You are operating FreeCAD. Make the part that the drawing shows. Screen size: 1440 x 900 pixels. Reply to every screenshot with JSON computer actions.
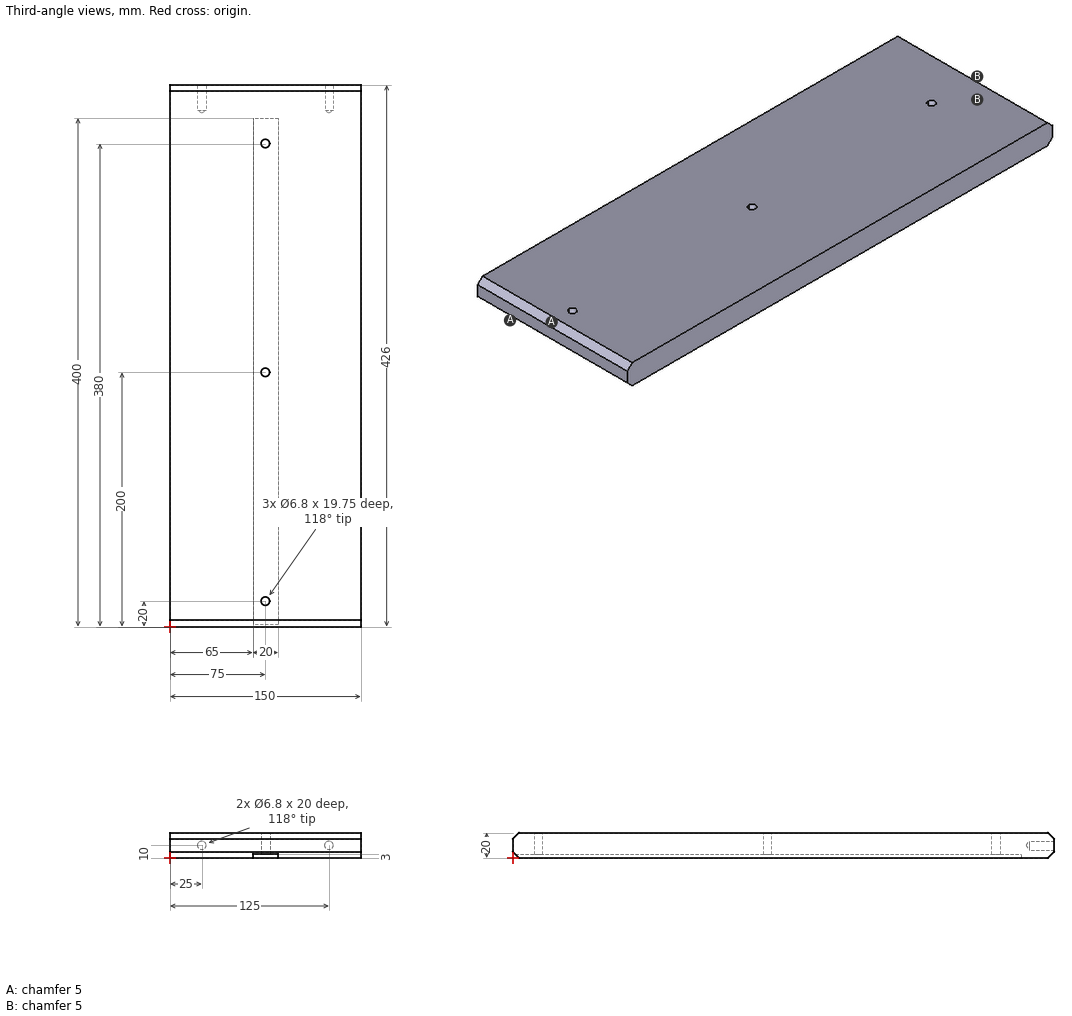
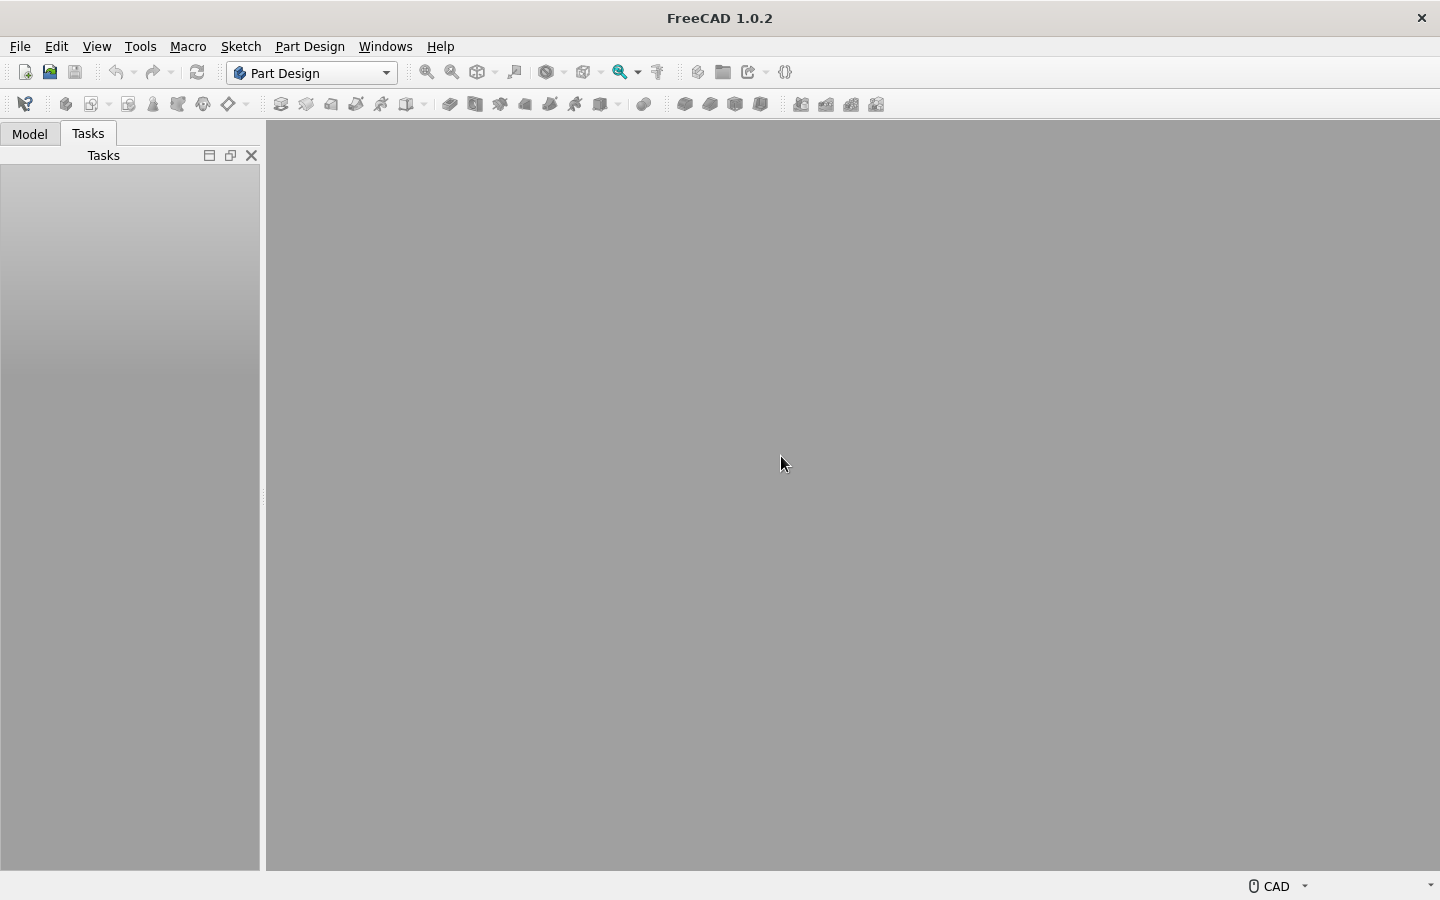
{"action": "left_click", "coordinate": [25, 72]}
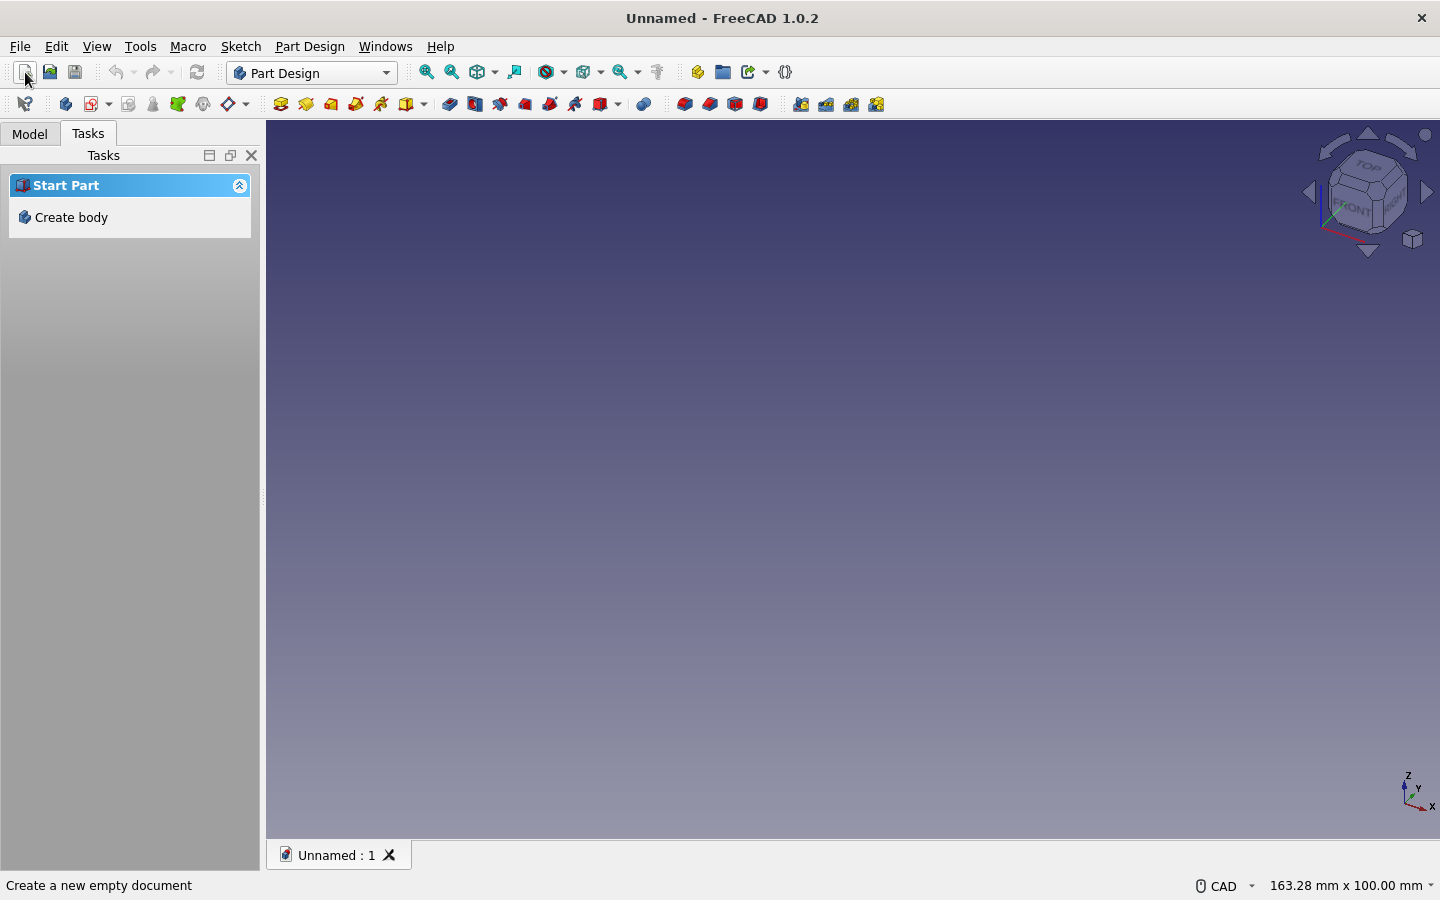
{"action": "left_click", "coordinate": [90, 104]}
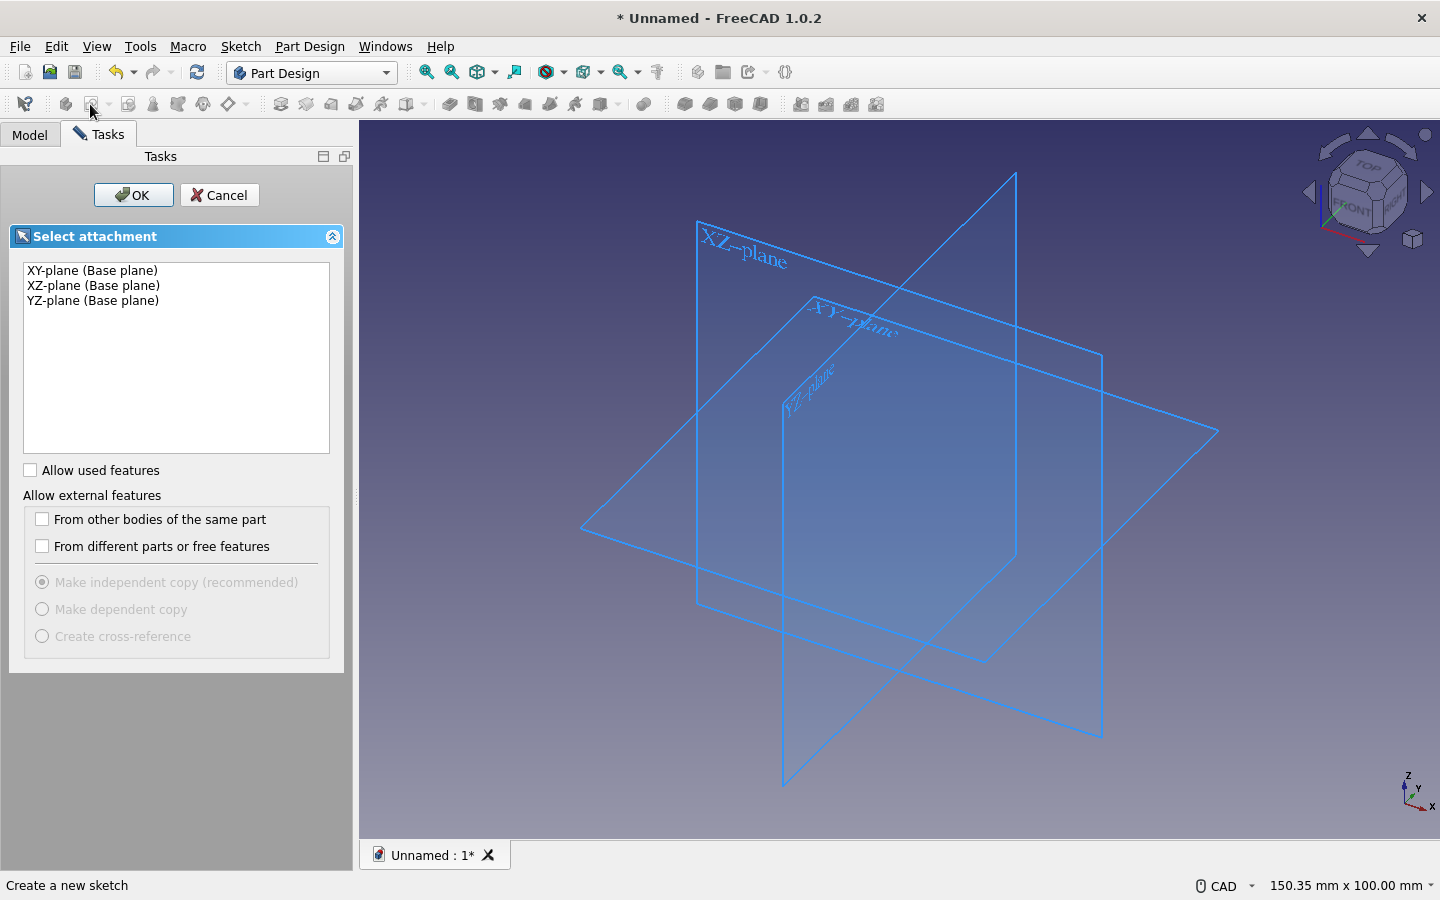
{"action": "left_click", "coordinate": [84, 270]}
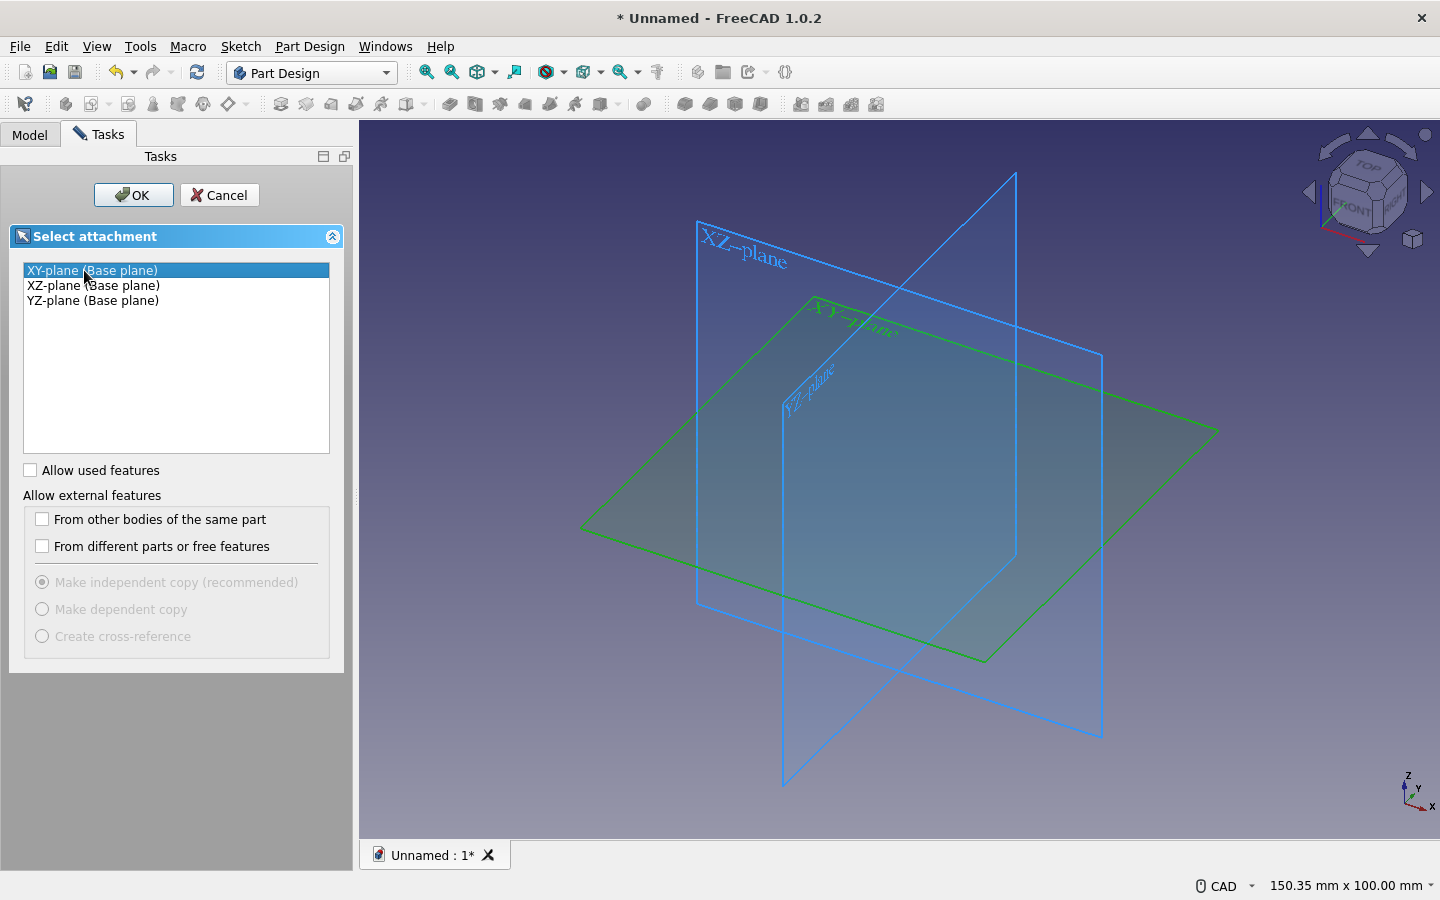
{"action": "left_click", "coordinate": [134, 195]}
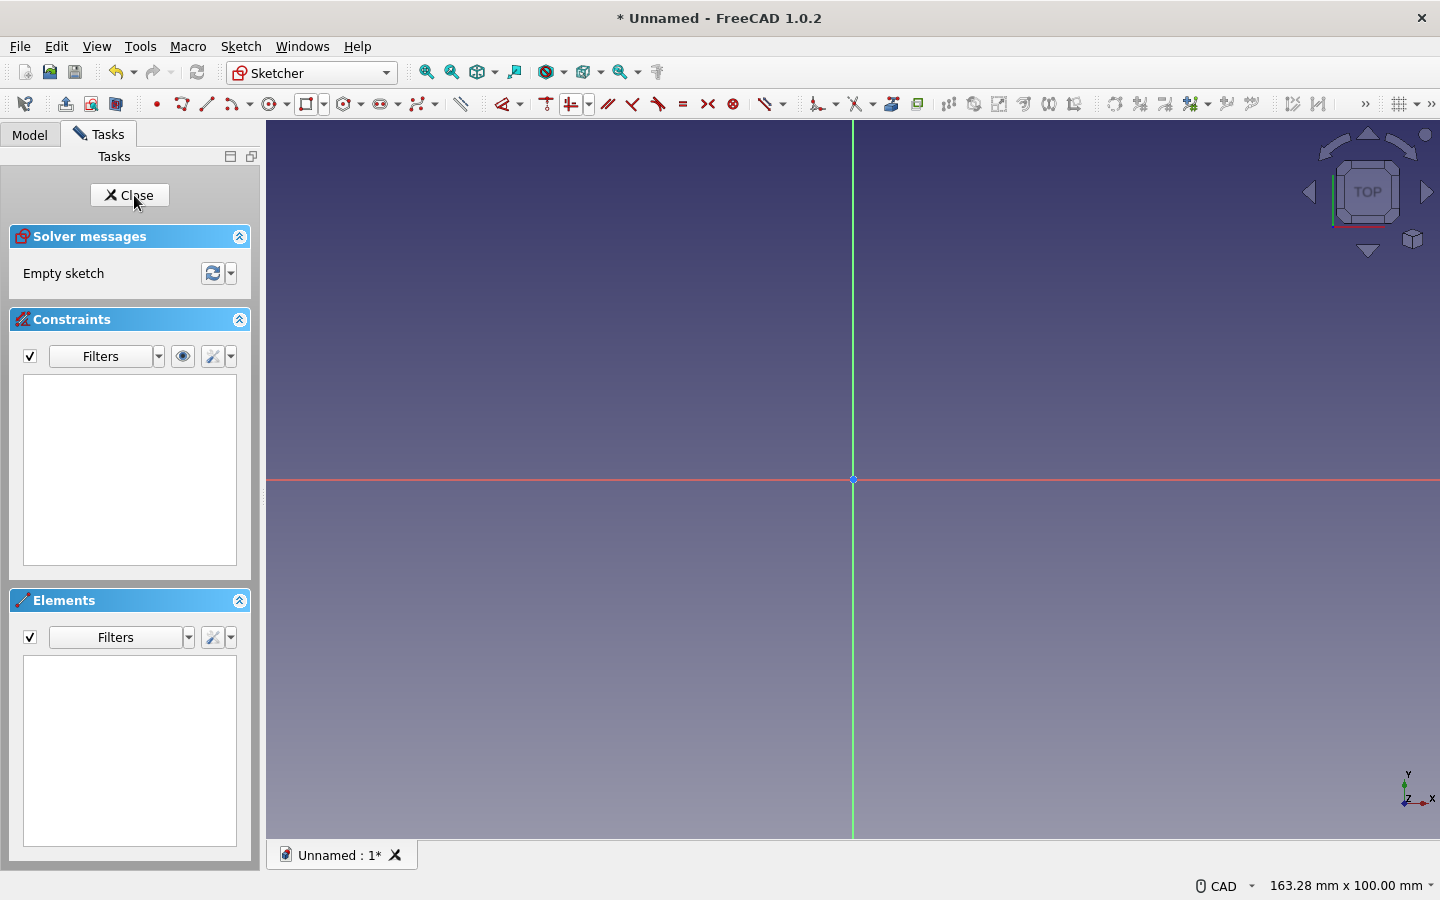
{"action": "scroll", "coordinate": [664, 783], "scroll_direction": "down", "scroll_amount": 9}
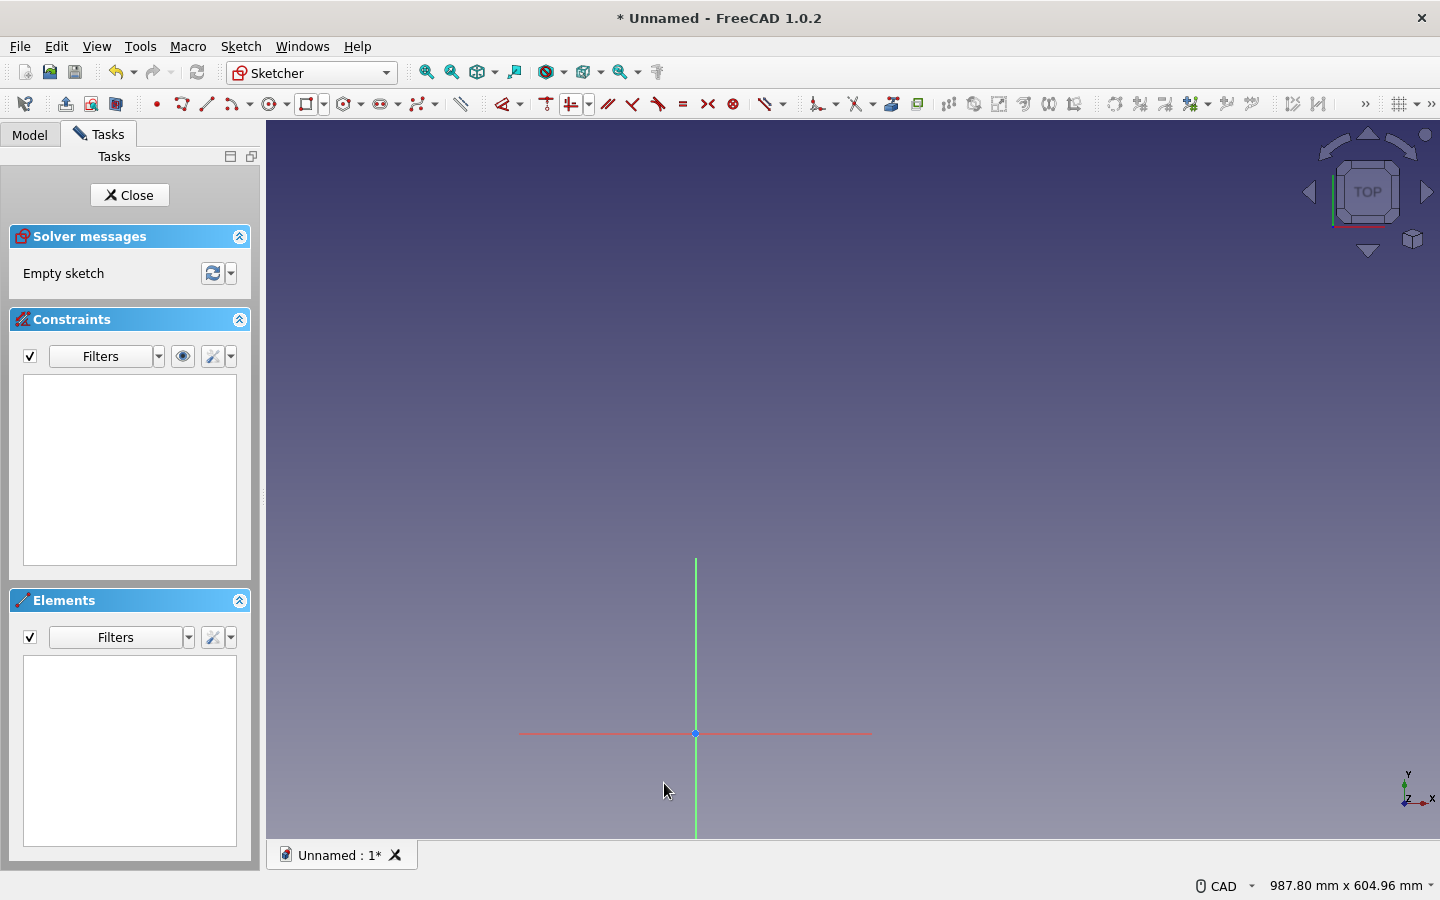
{"action": "left_click", "coordinate": [306, 104]}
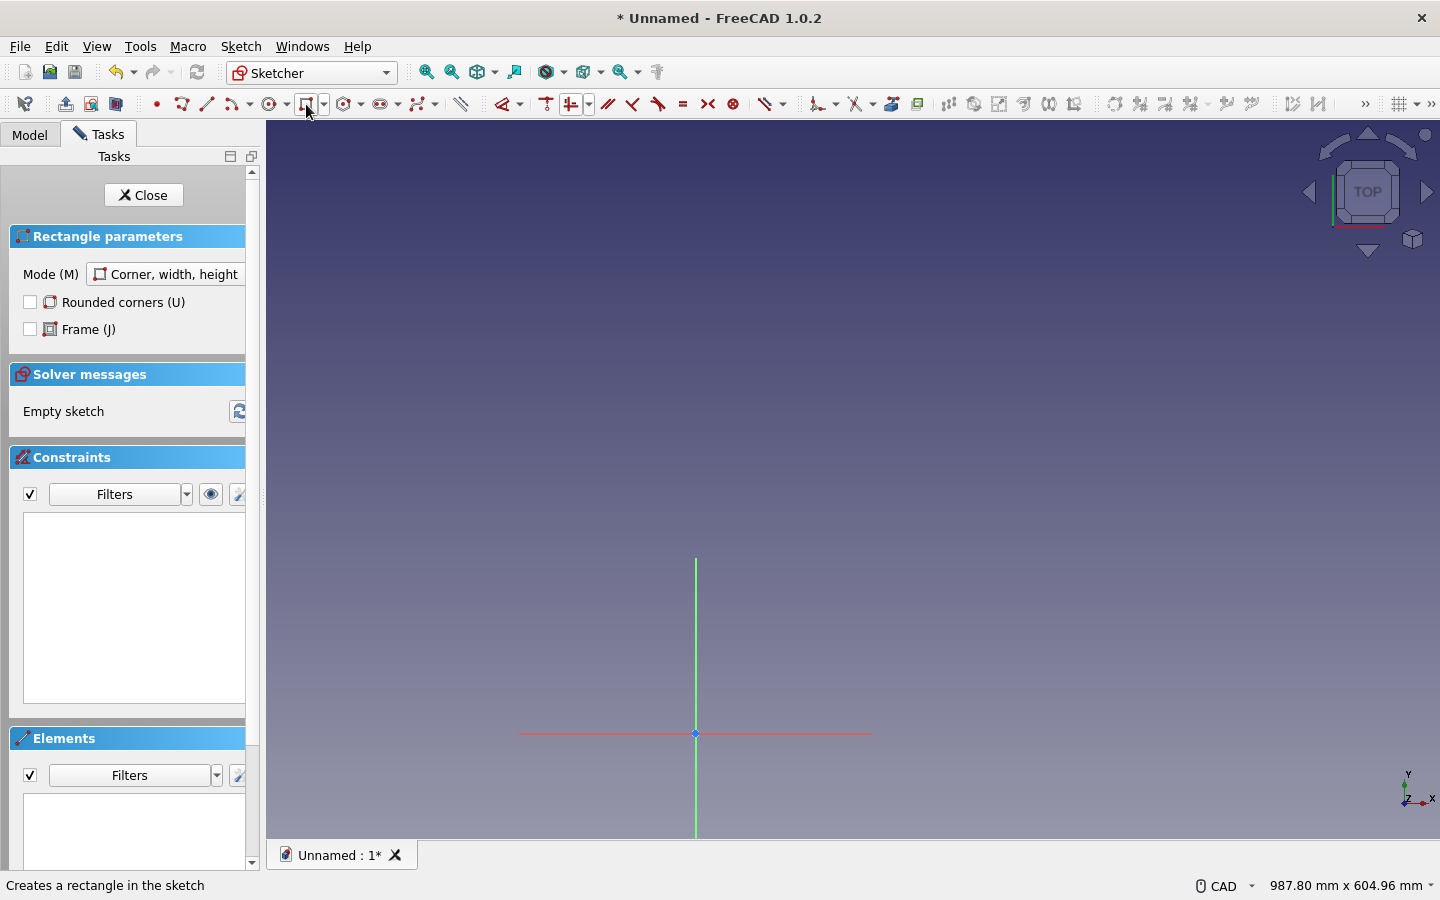
{"action": "left_click", "coordinate": [696, 734]}
{"action": "left_click", "coordinate": [874, 227]}
{"action": "key", "text": "Escape"}